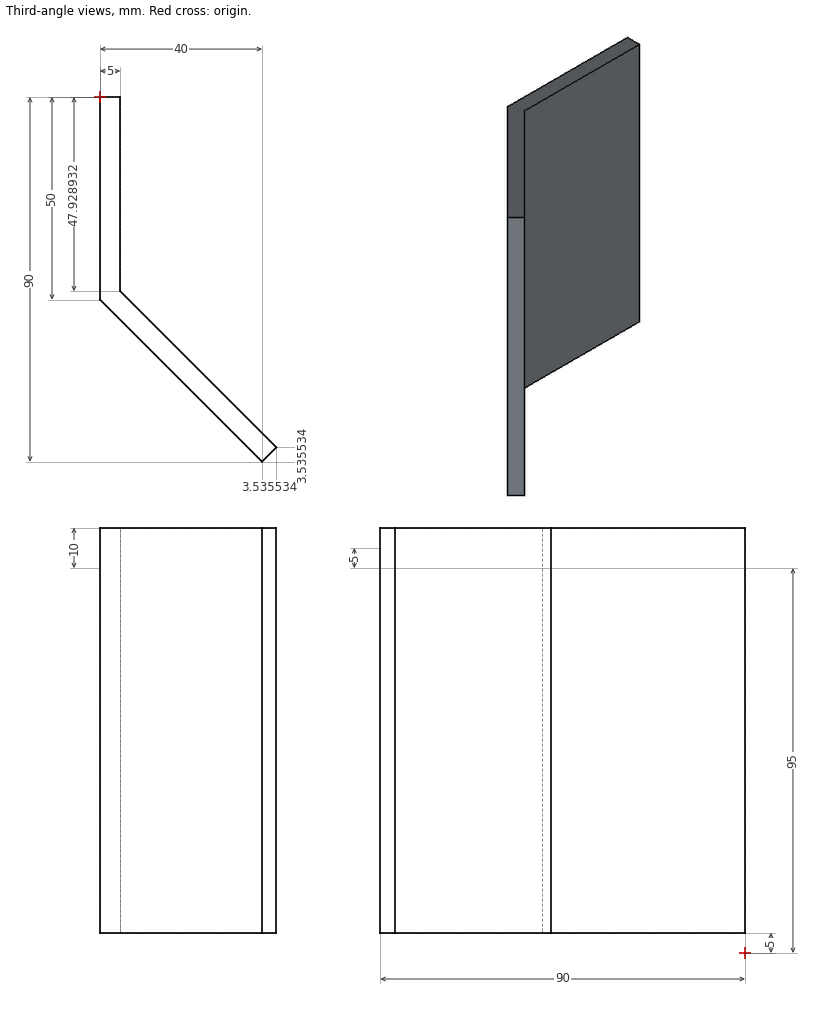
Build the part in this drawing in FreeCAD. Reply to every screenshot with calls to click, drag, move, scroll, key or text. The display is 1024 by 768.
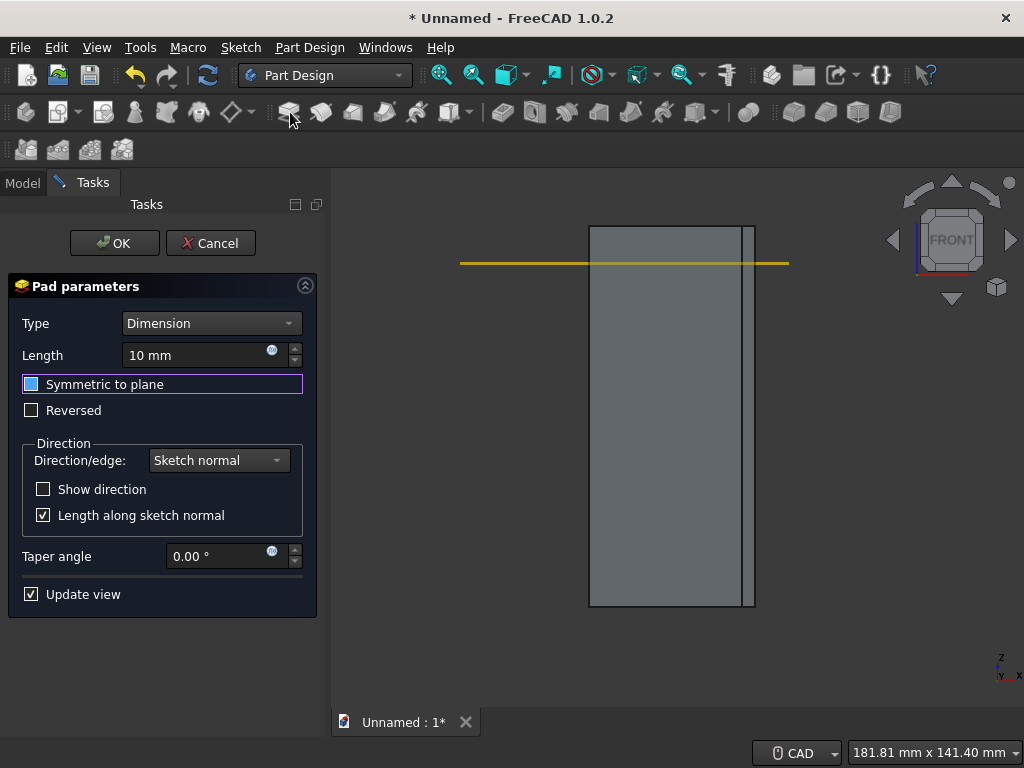
click(115, 243)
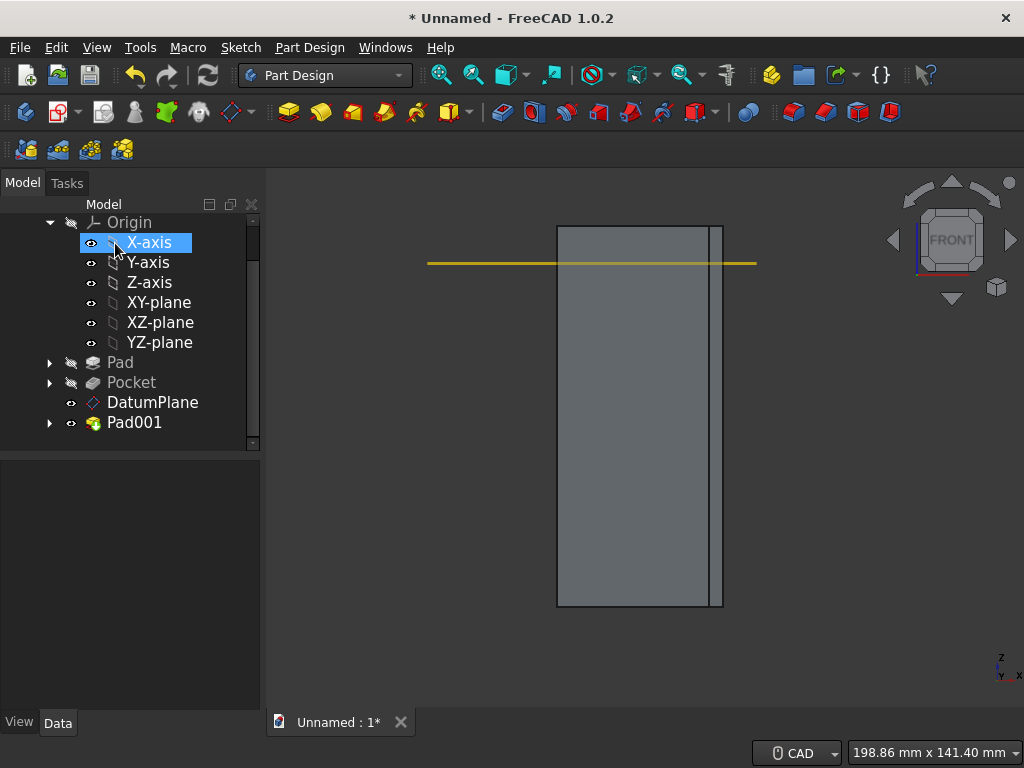
click(116, 403)
key(space)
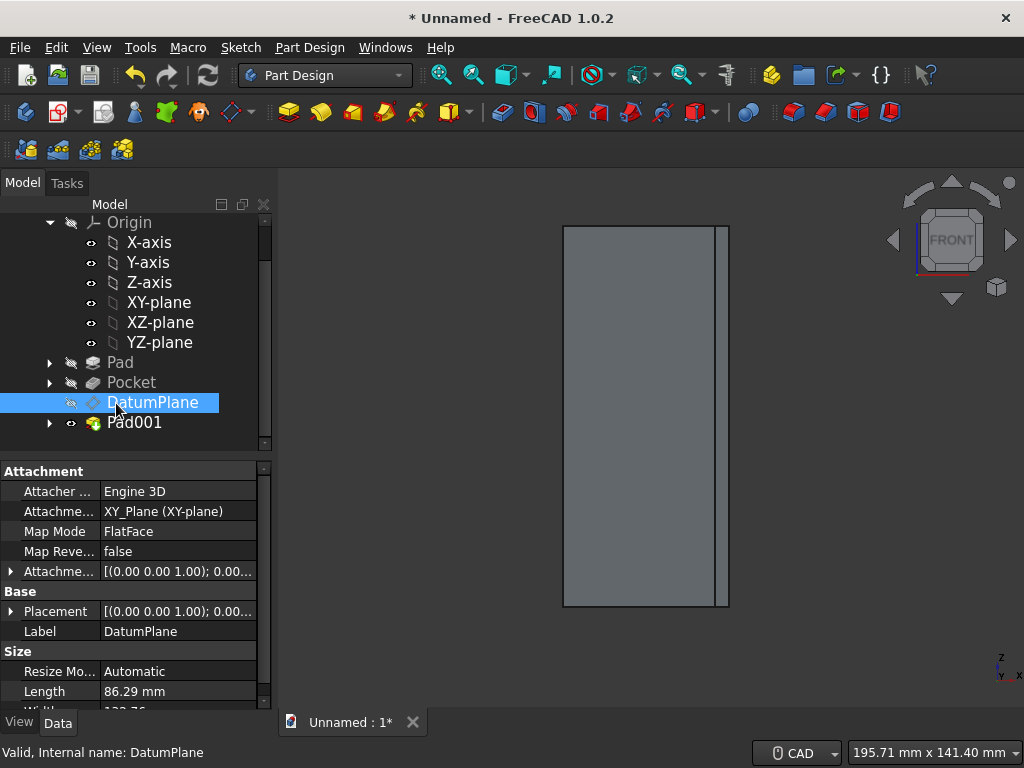
key(0)